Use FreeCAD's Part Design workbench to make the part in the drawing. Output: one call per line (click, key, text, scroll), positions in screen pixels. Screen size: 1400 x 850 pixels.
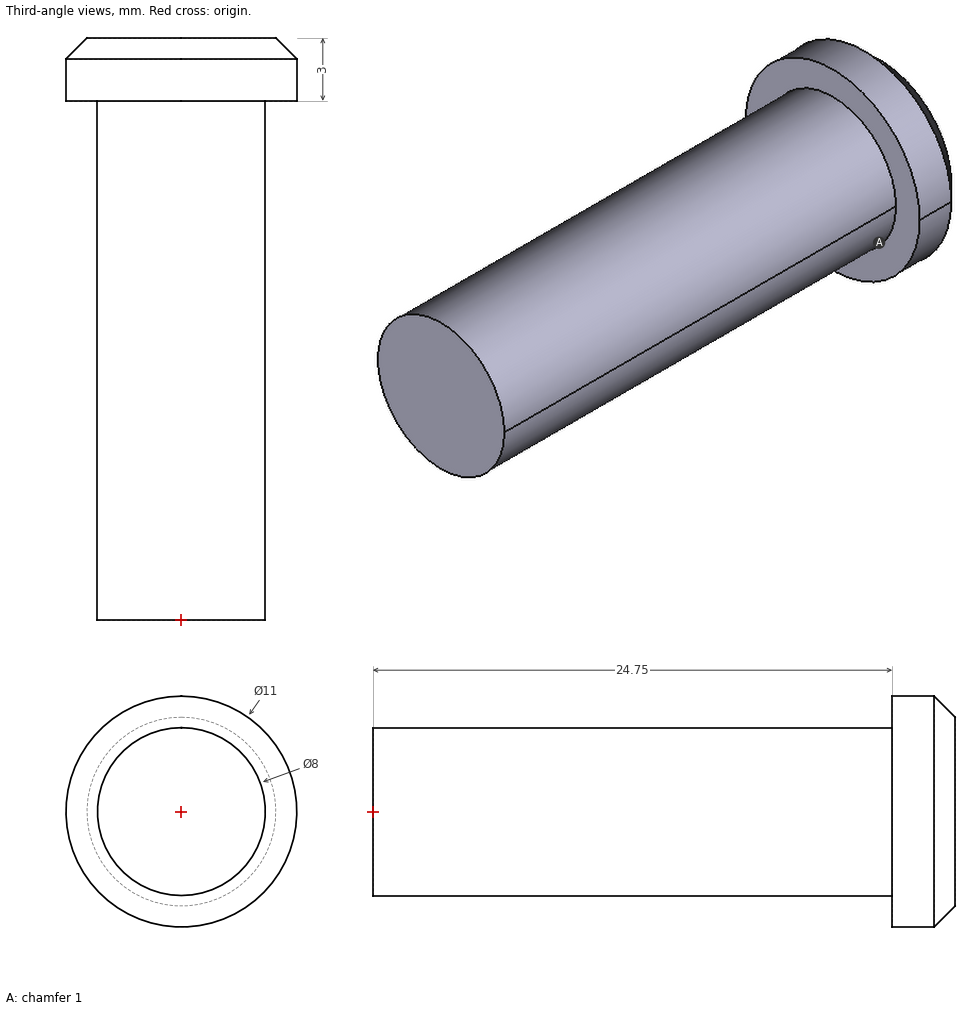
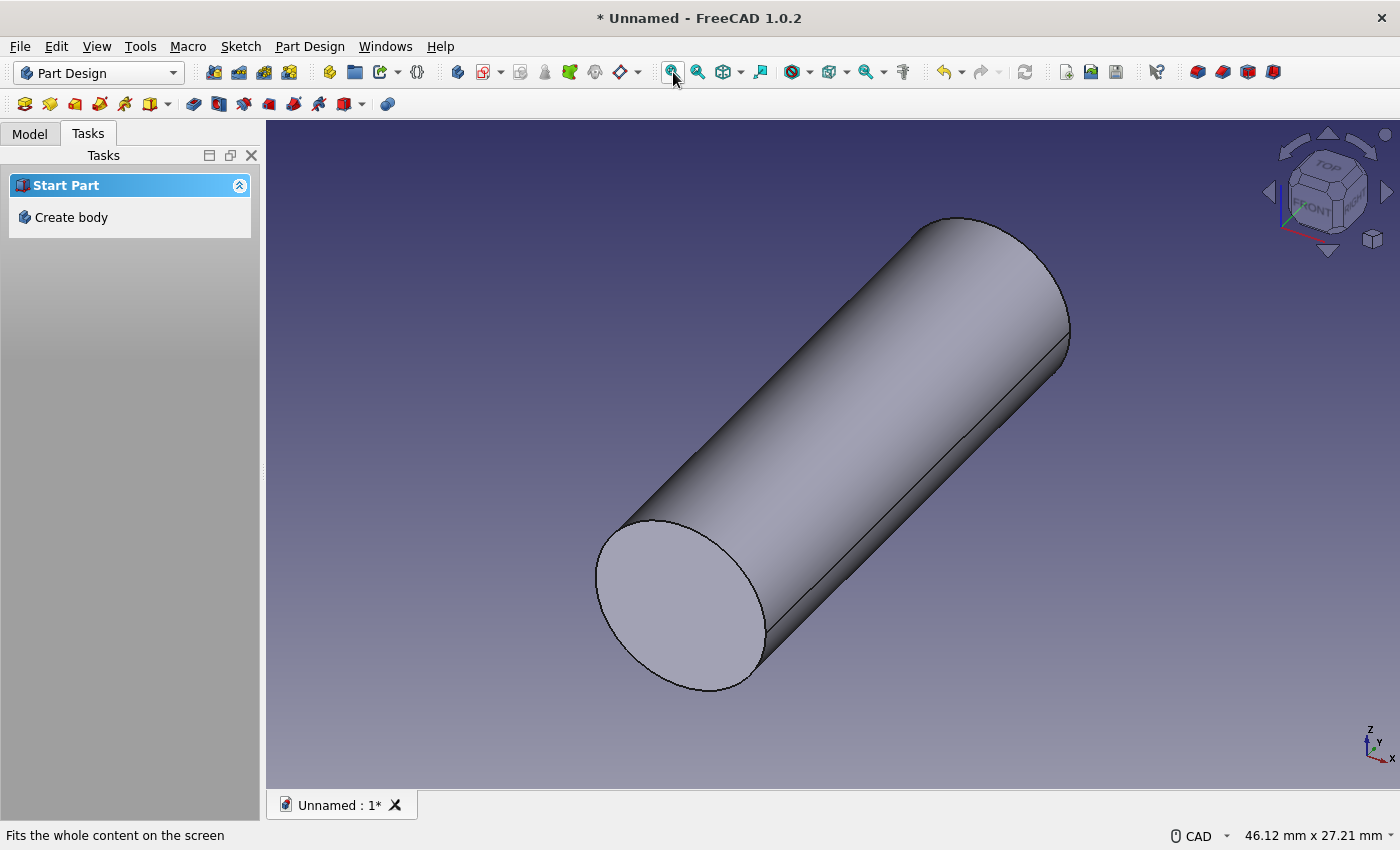
key(4)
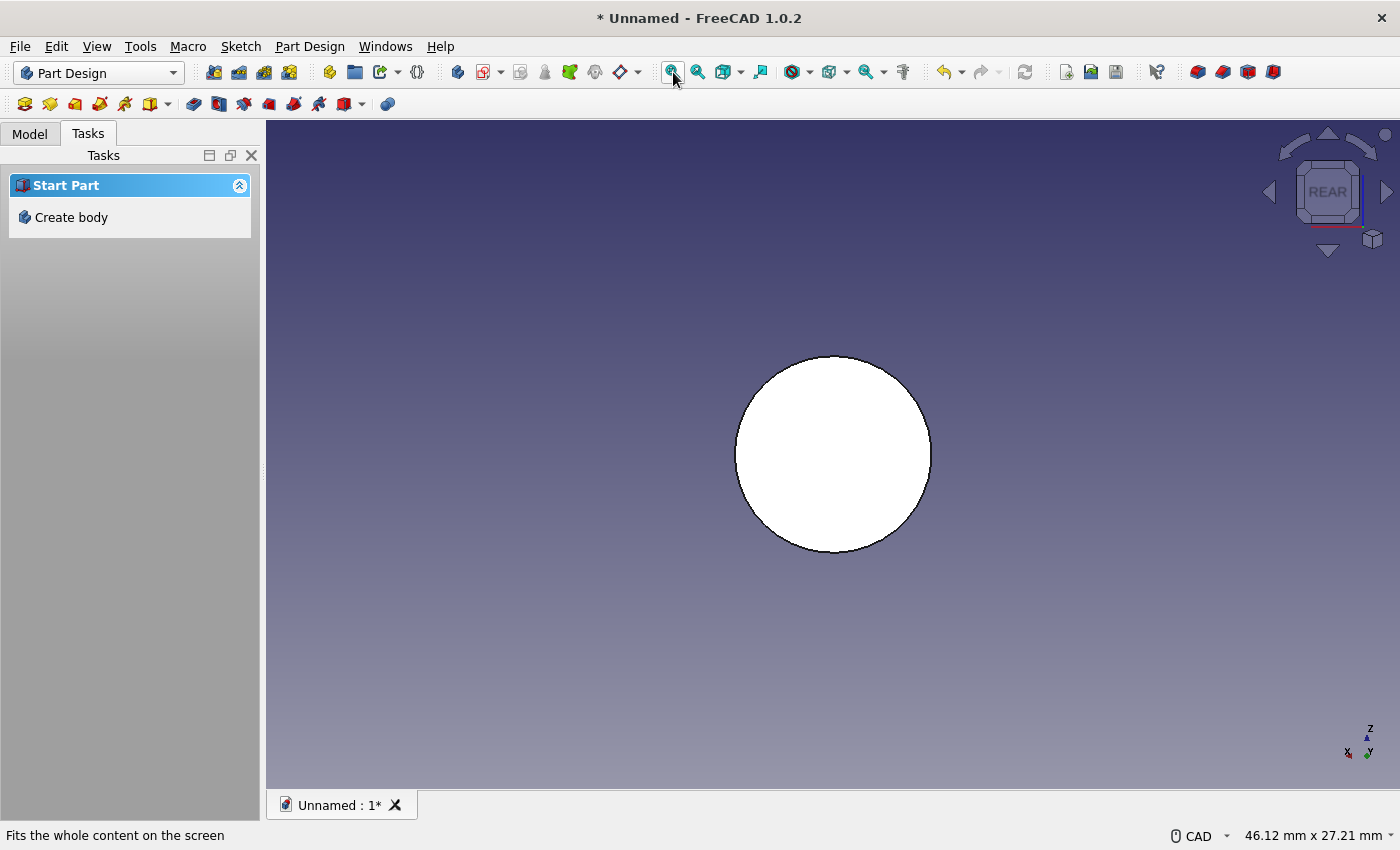
click(673, 72)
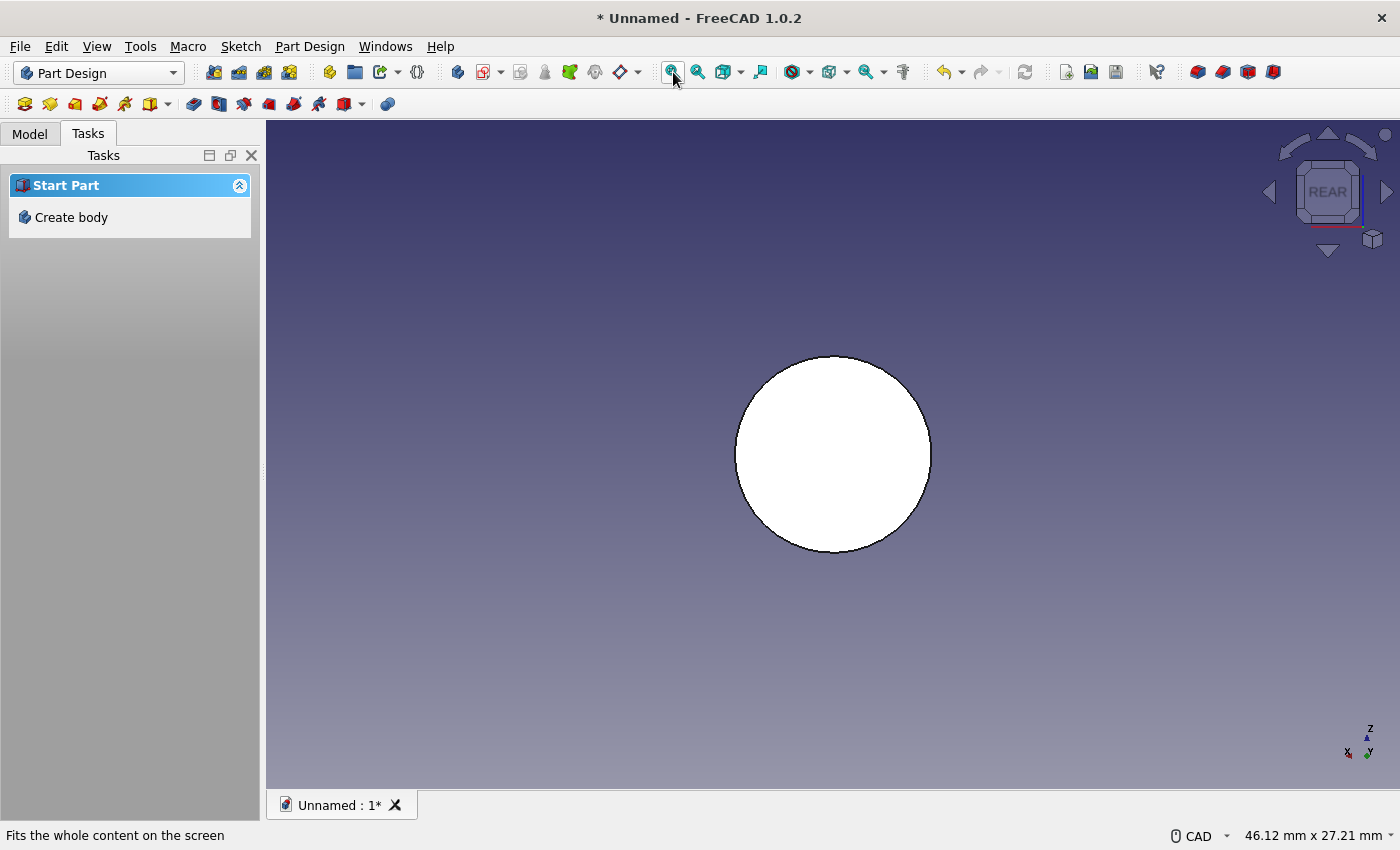
click(833, 454)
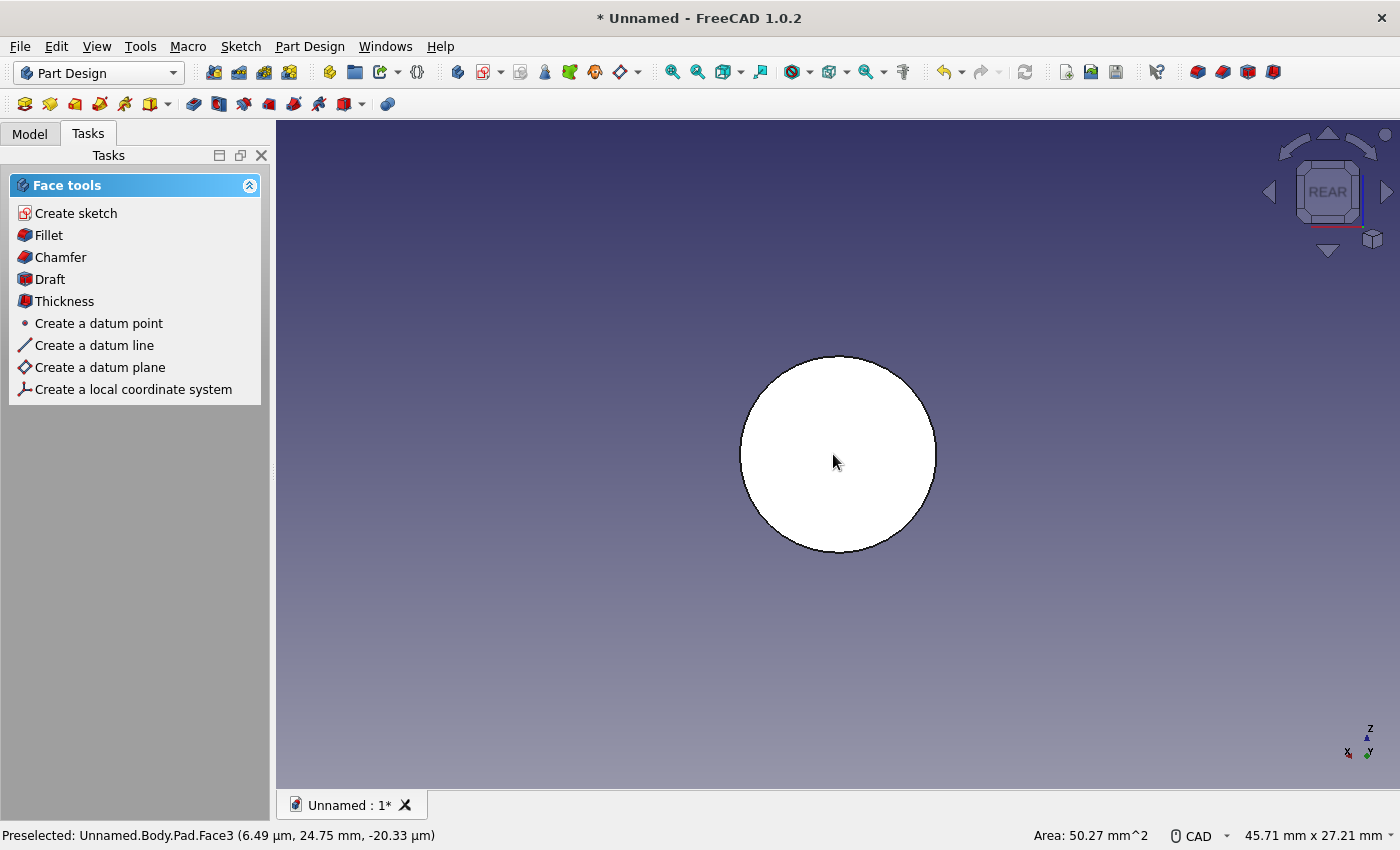
click(482, 72)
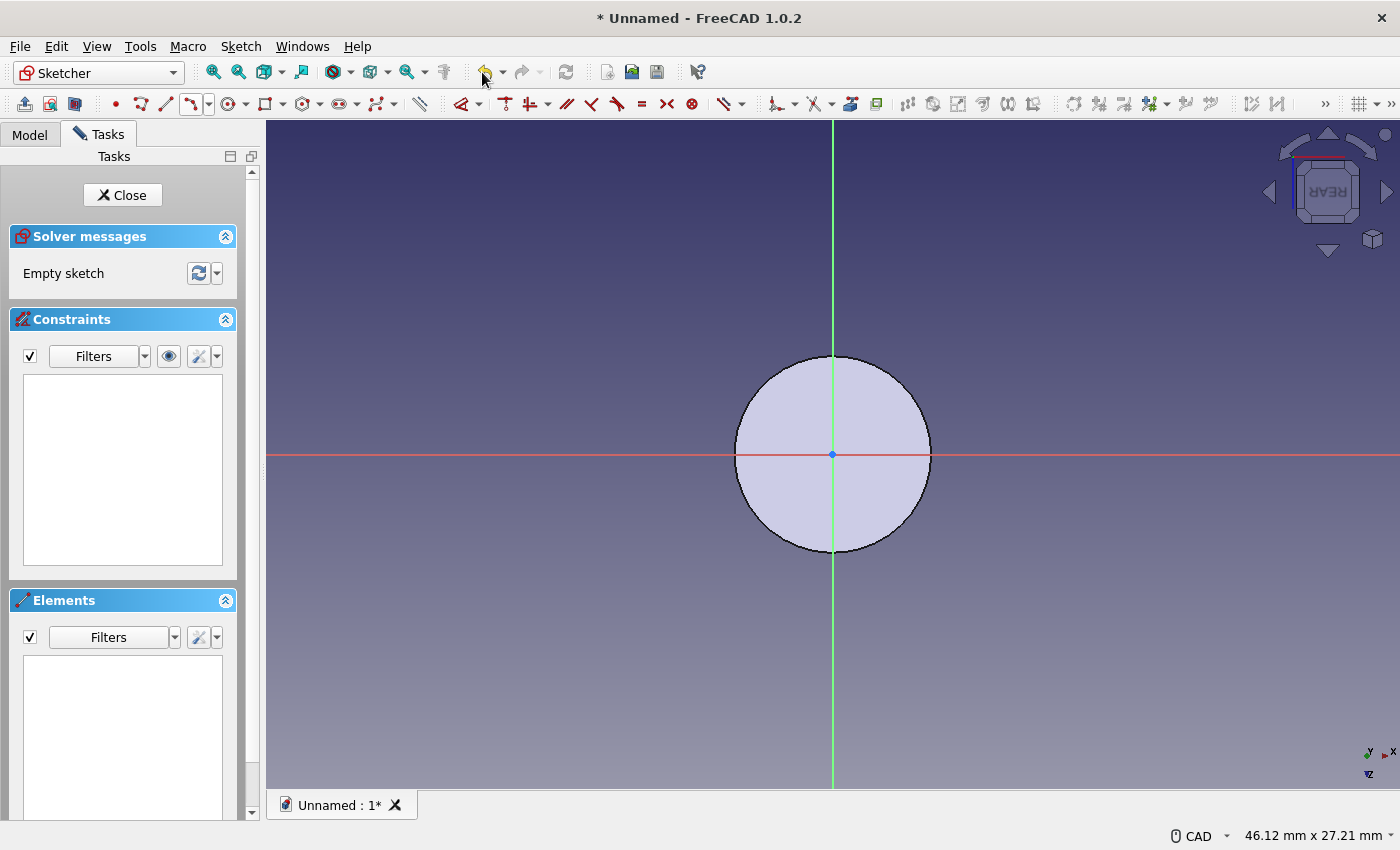
scroll(972, 454, up, 2)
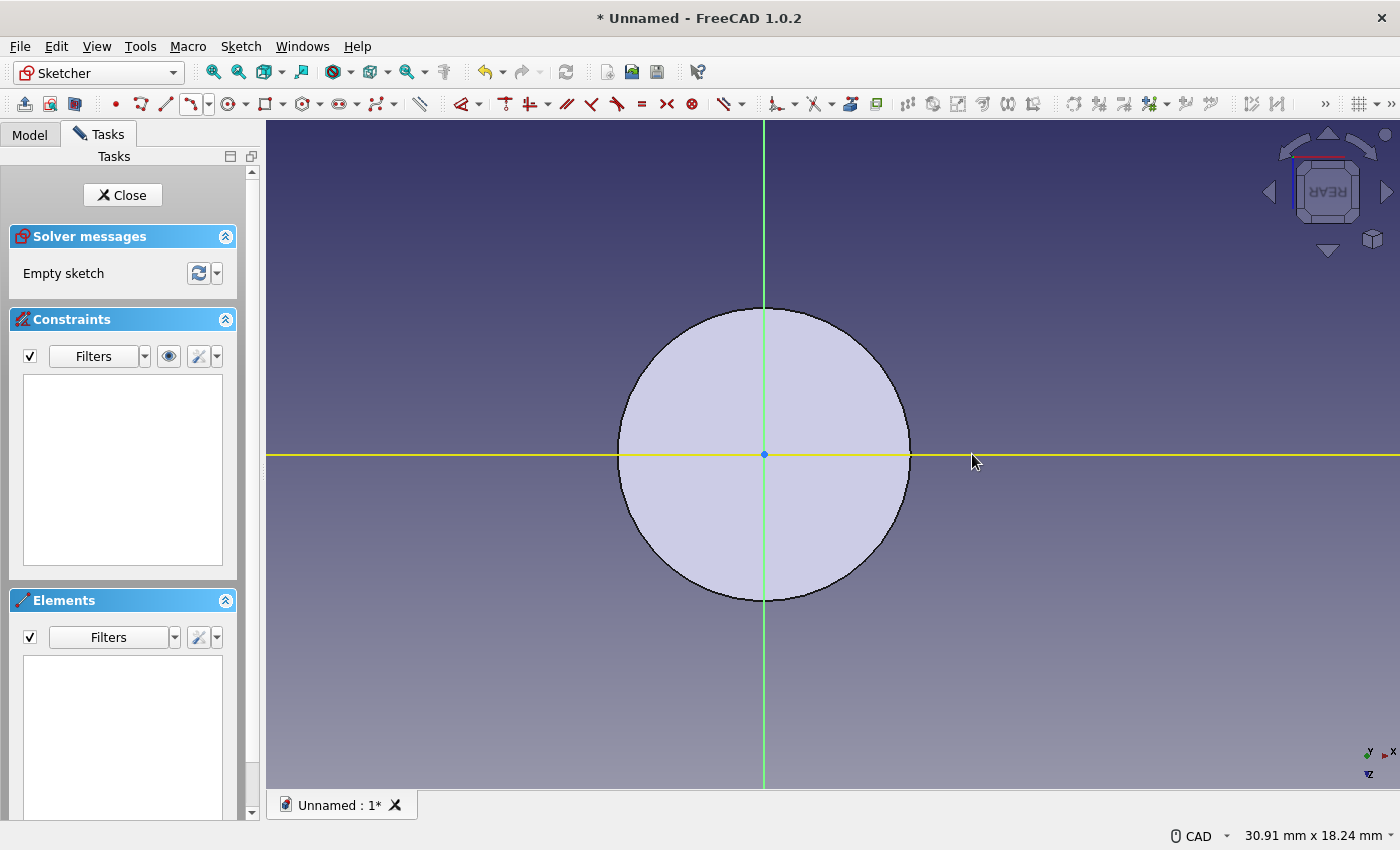
click(228, 104)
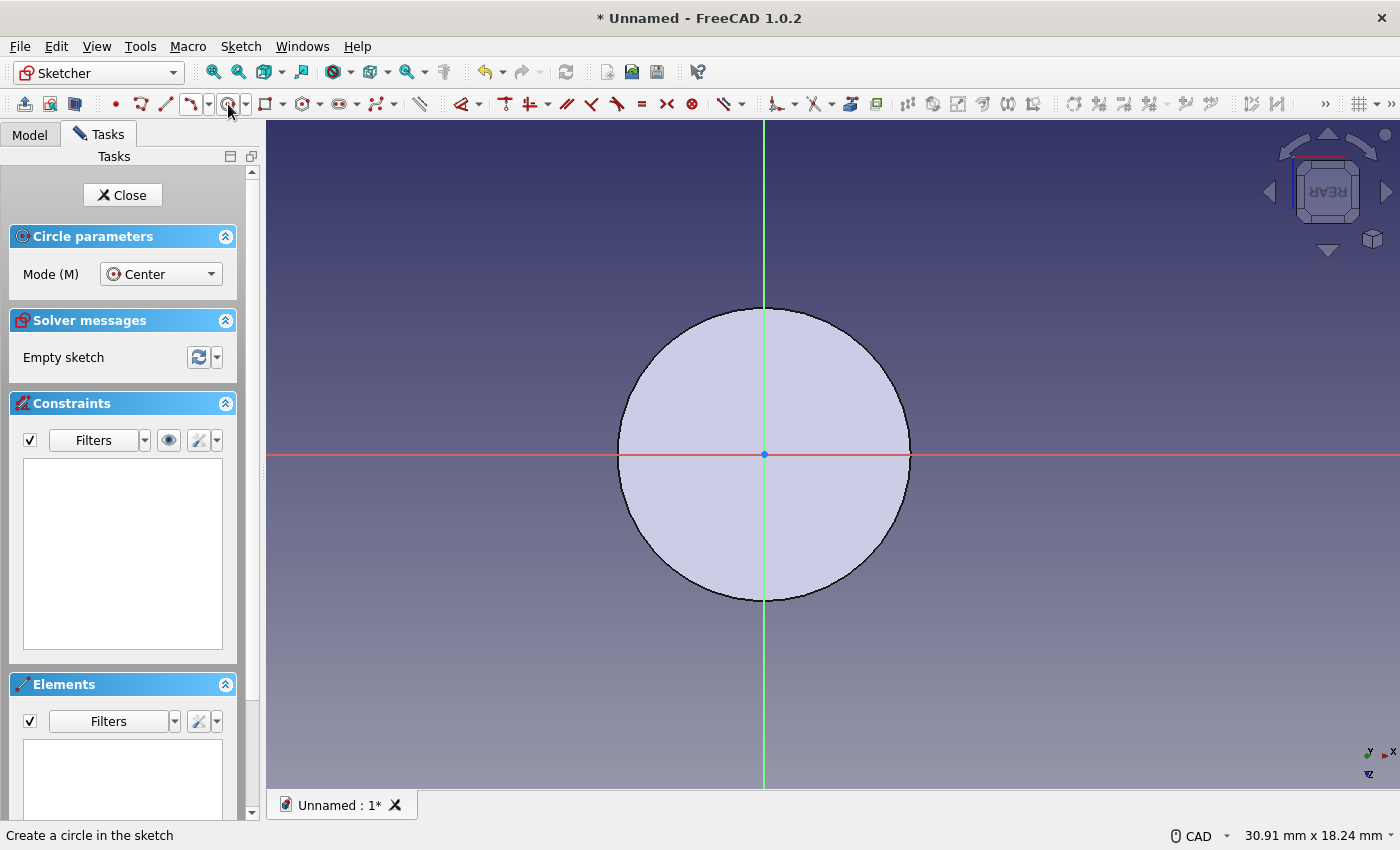
click(764, 454)
click(907, 312)
key(Escape)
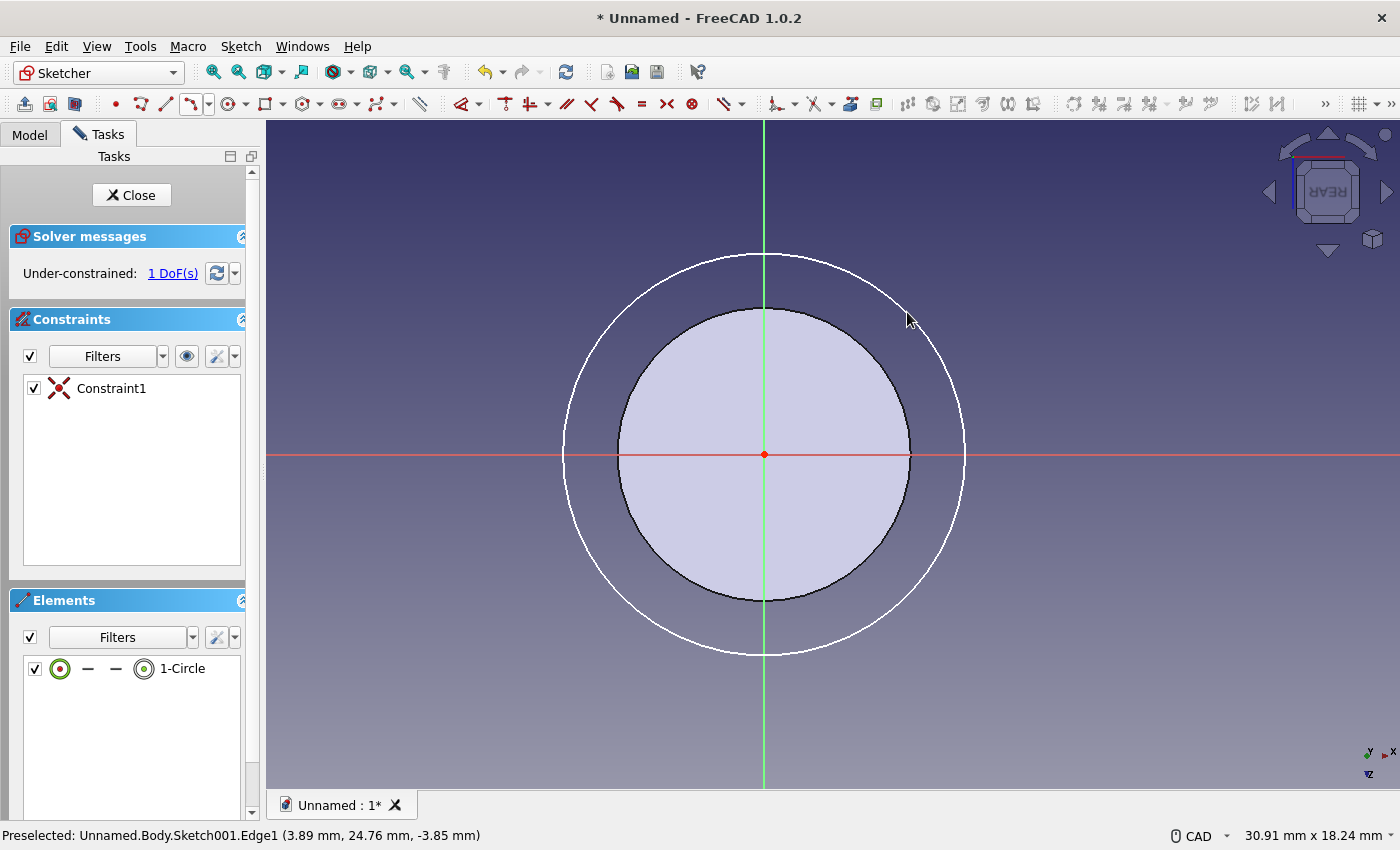
click(460, 104)